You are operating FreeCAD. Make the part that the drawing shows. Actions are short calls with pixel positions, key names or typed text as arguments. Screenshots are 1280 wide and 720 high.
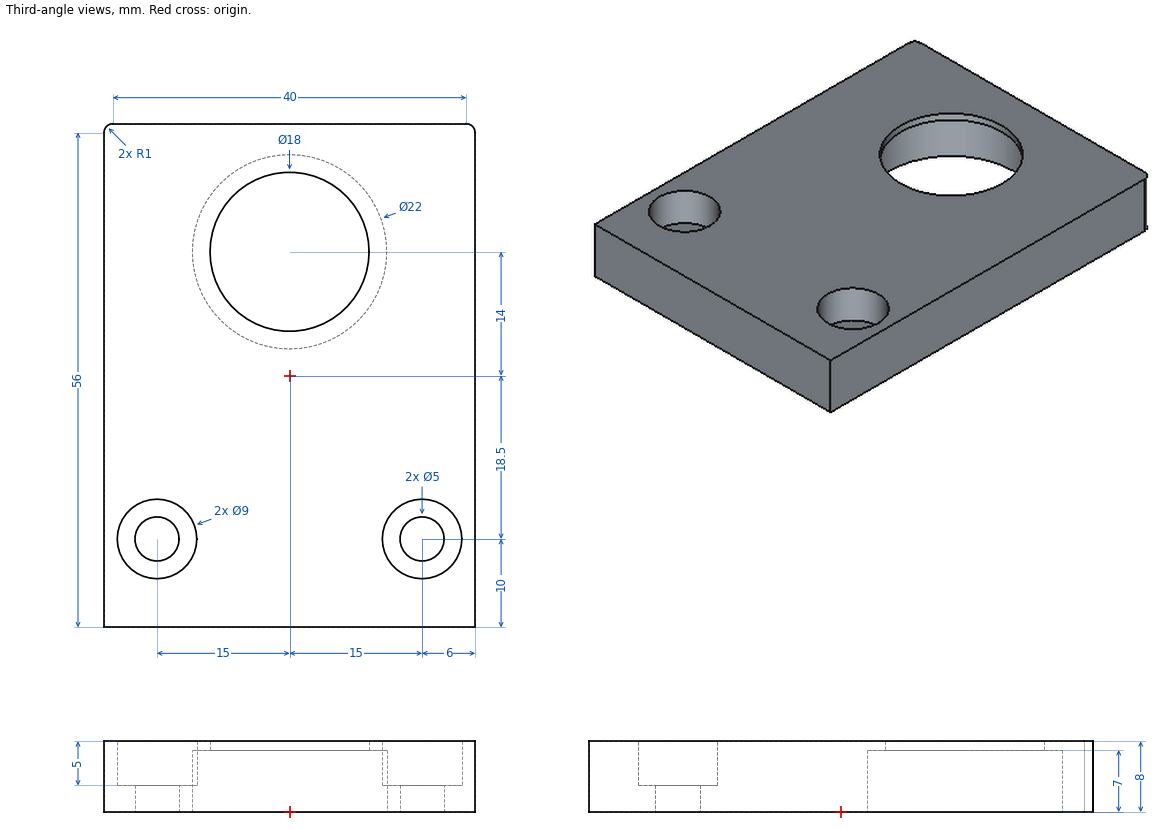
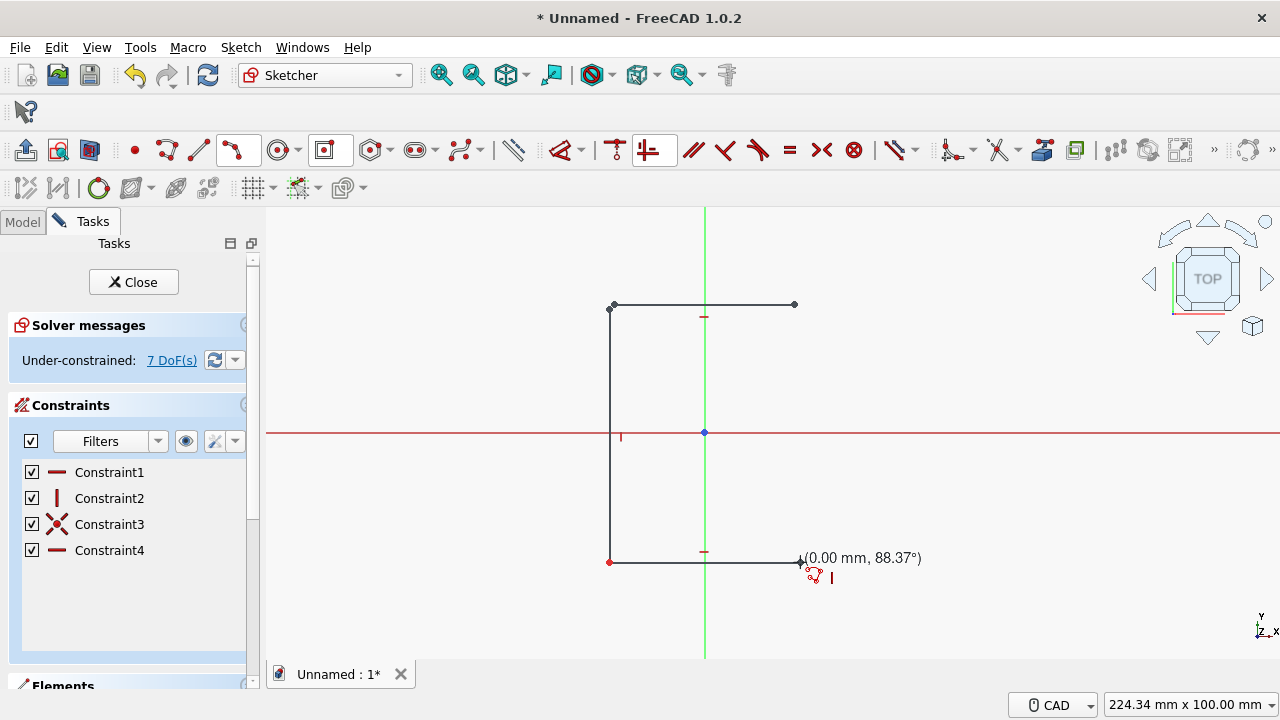
scroll(800, 309, up, 5)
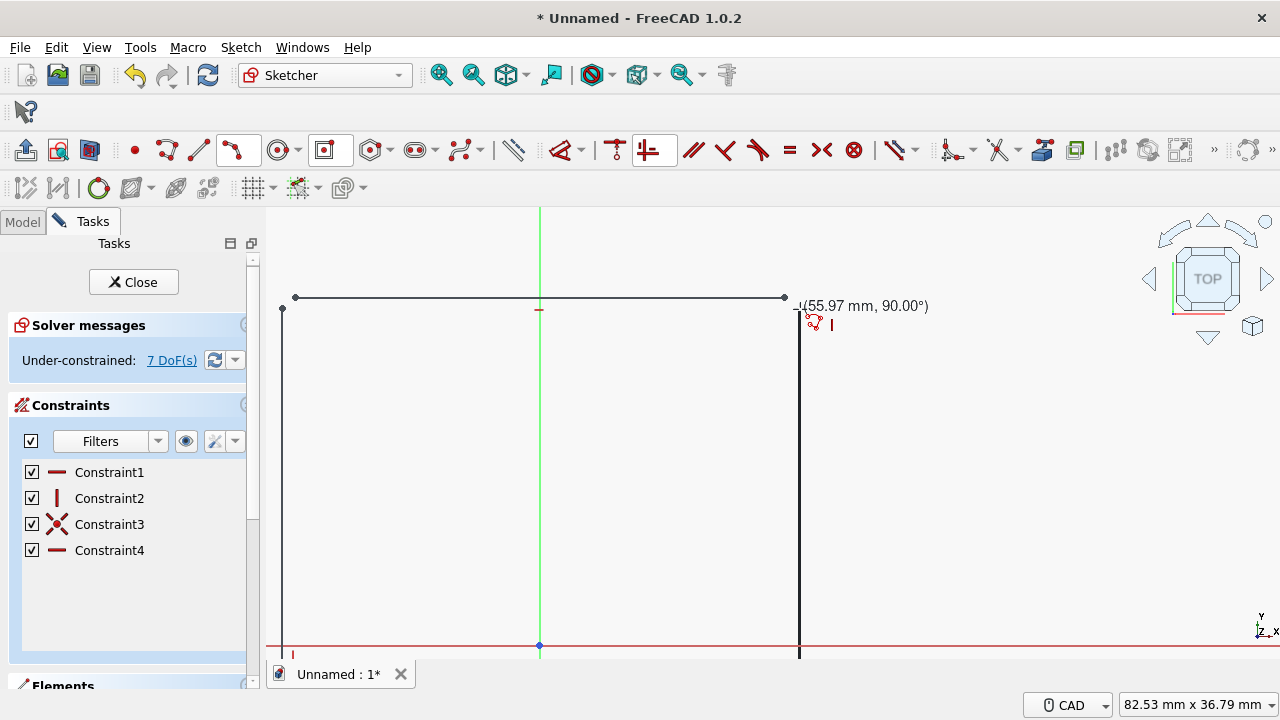
click(799, 308)
right_click(799, 308)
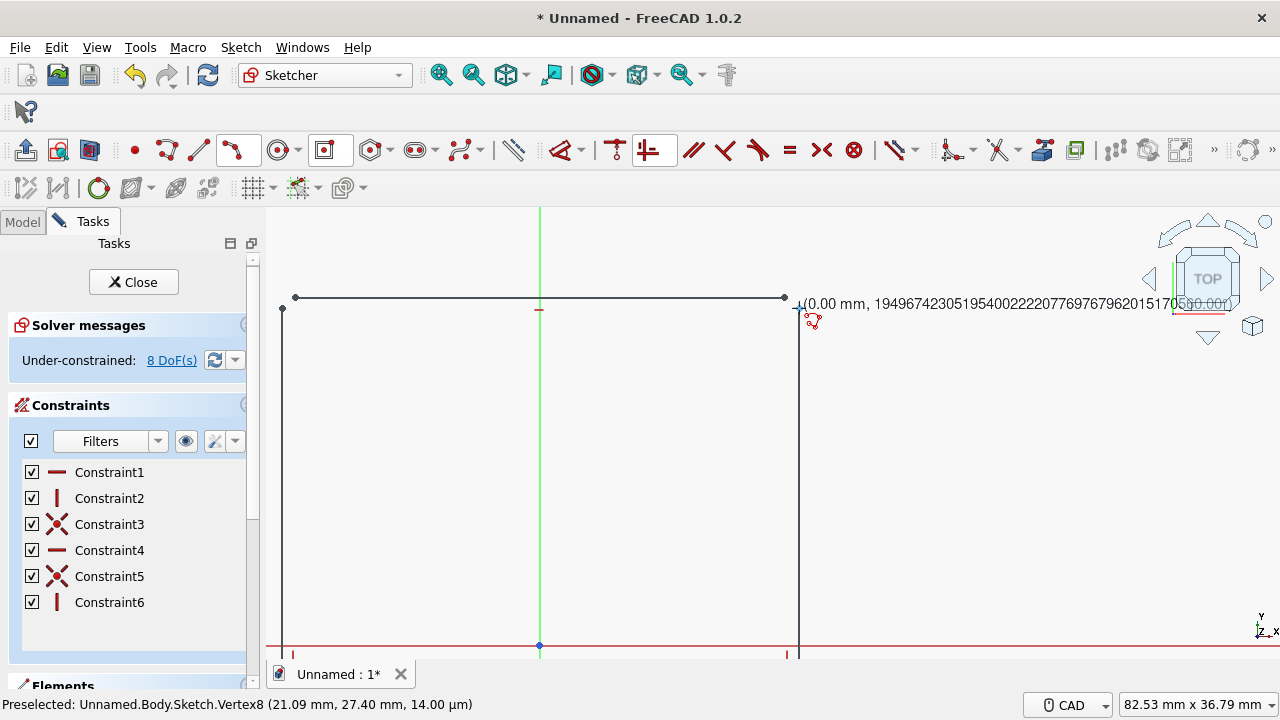
click(232, 150)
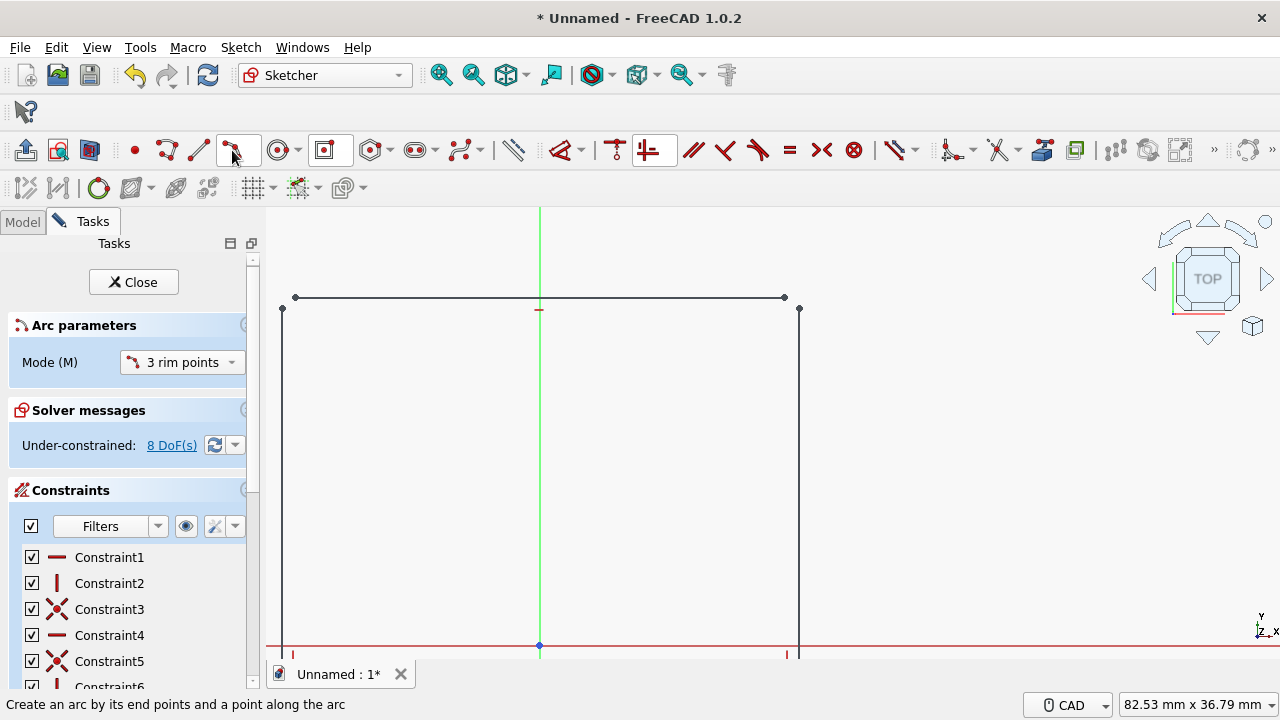
click(295, 298)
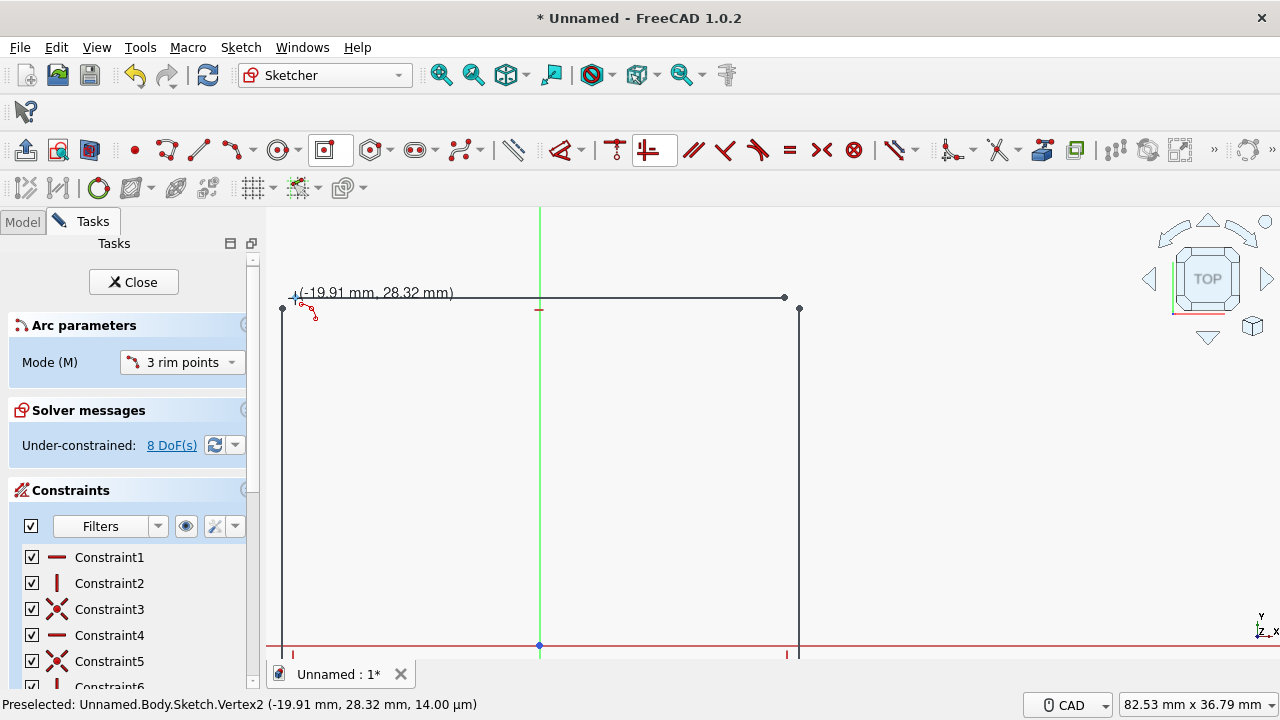
scroll(800, 309, down, 5)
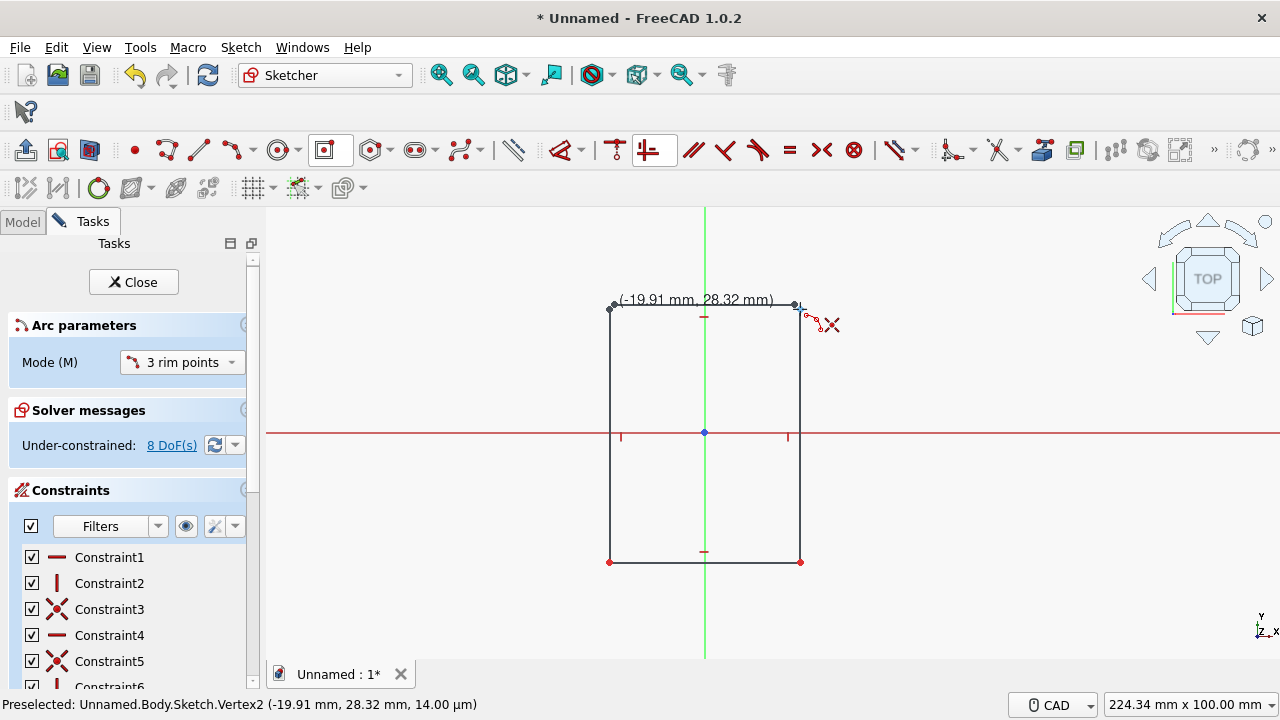
scroll(610, 309, up, 5)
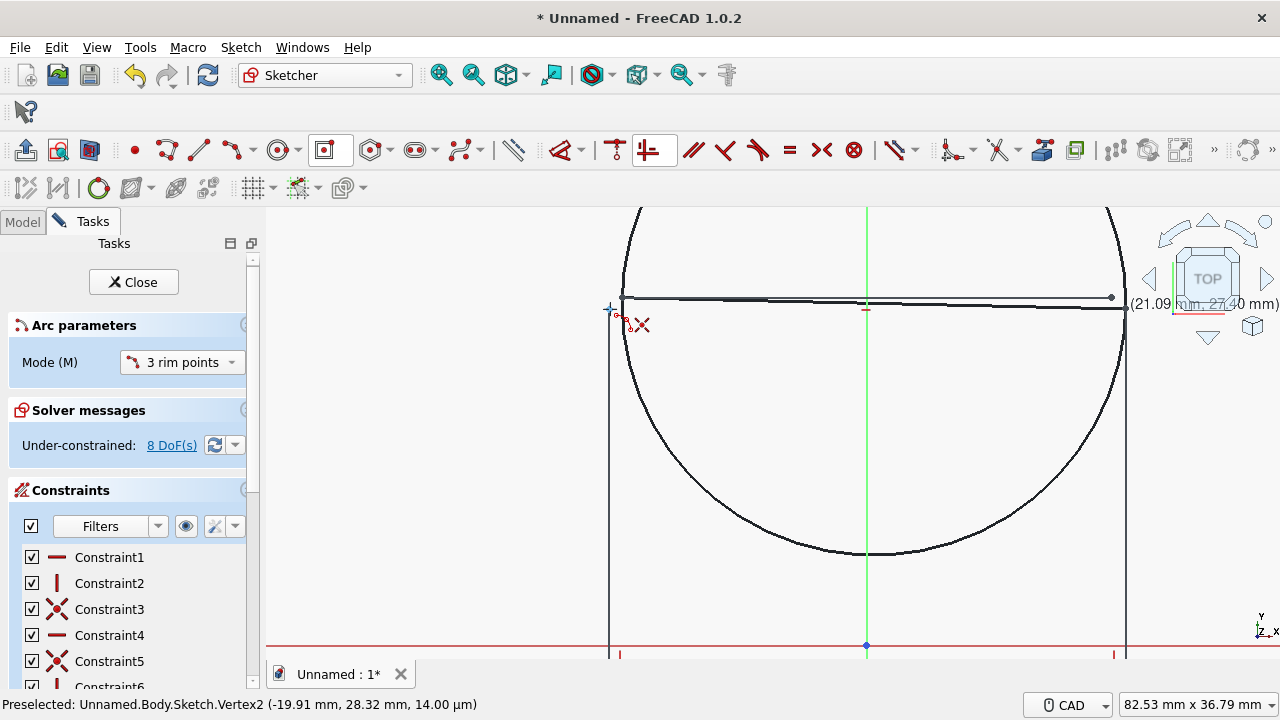
click(609, 309)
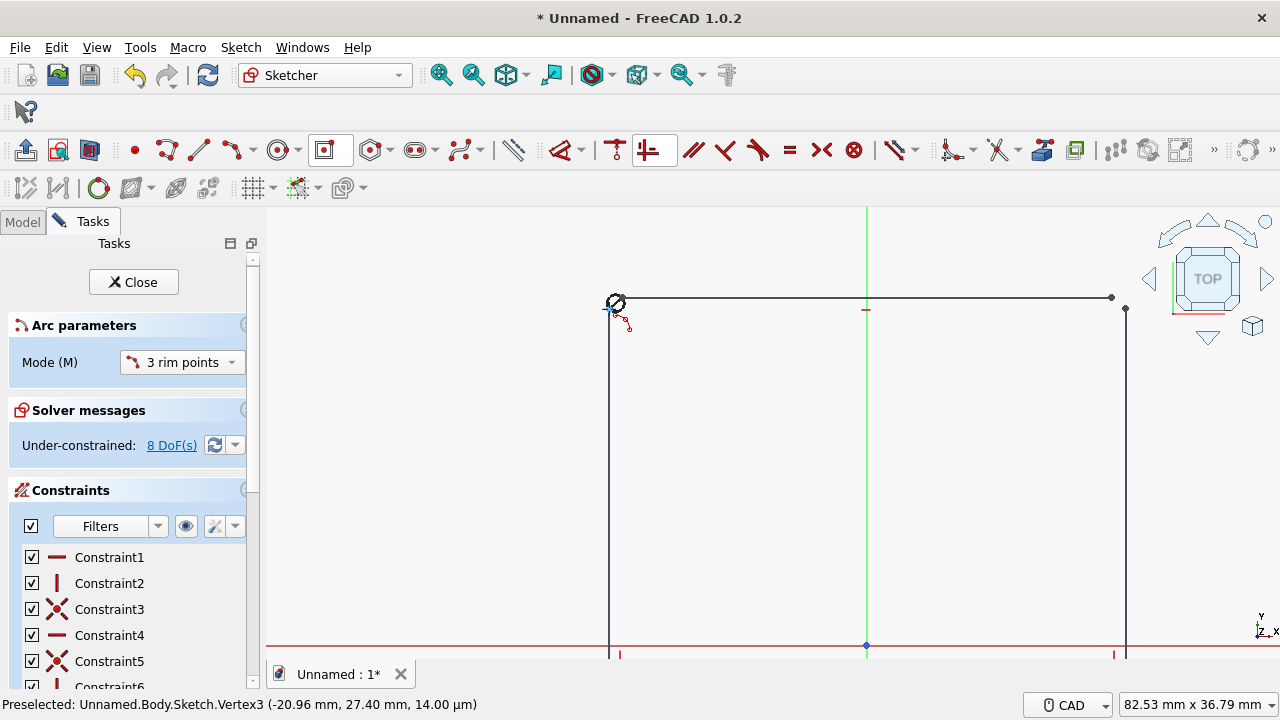
scroll(612, 299, up, 8)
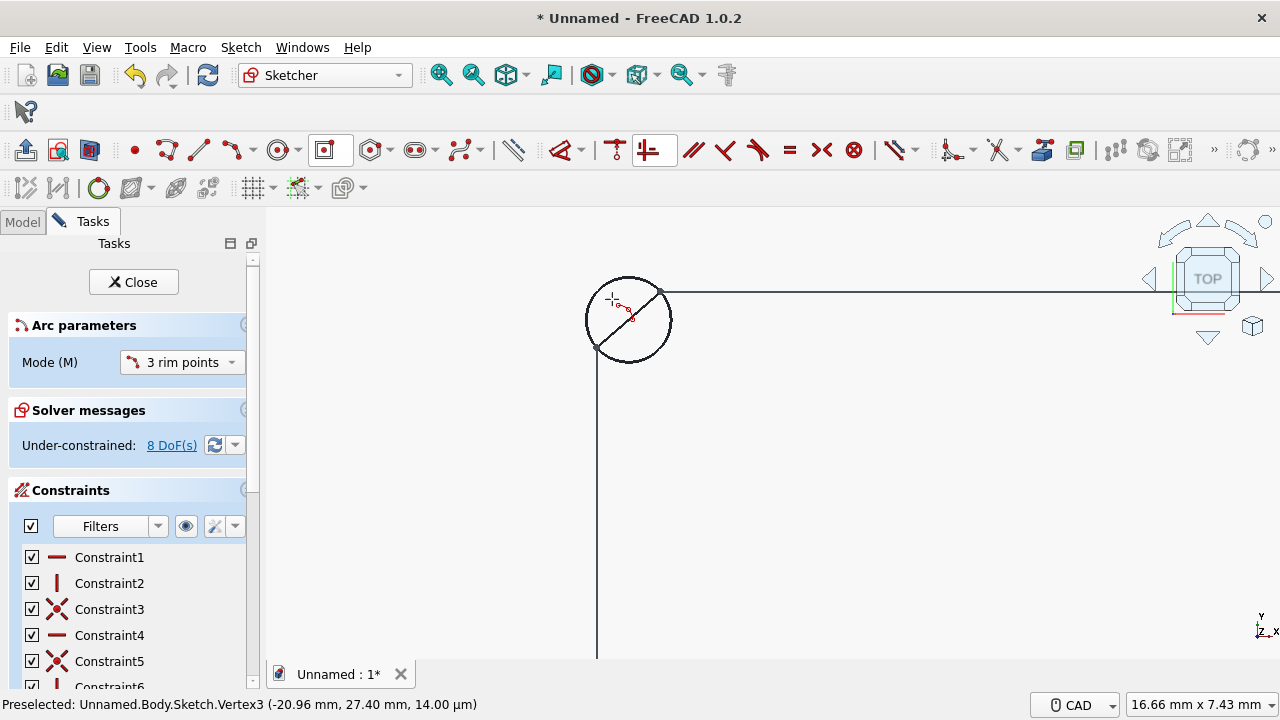
click(612, 299)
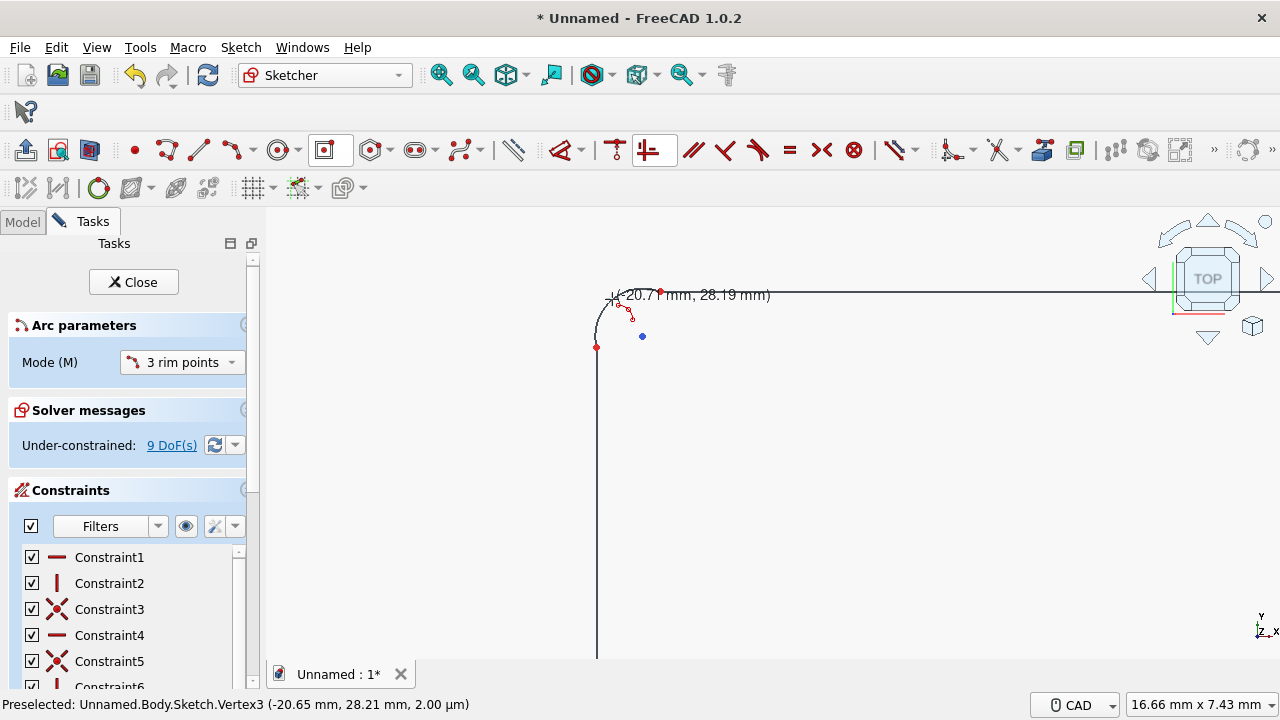
scroll(611, 306, down, 13)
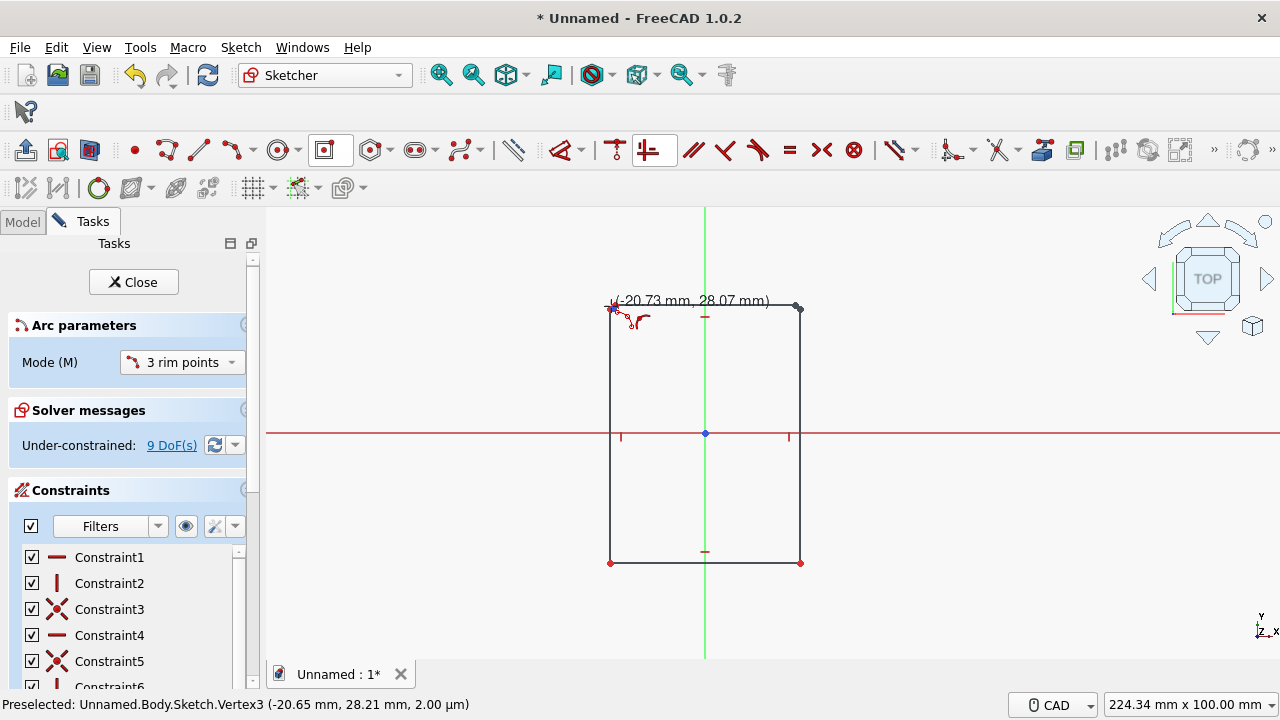
scroll(800, 309, up, 5)